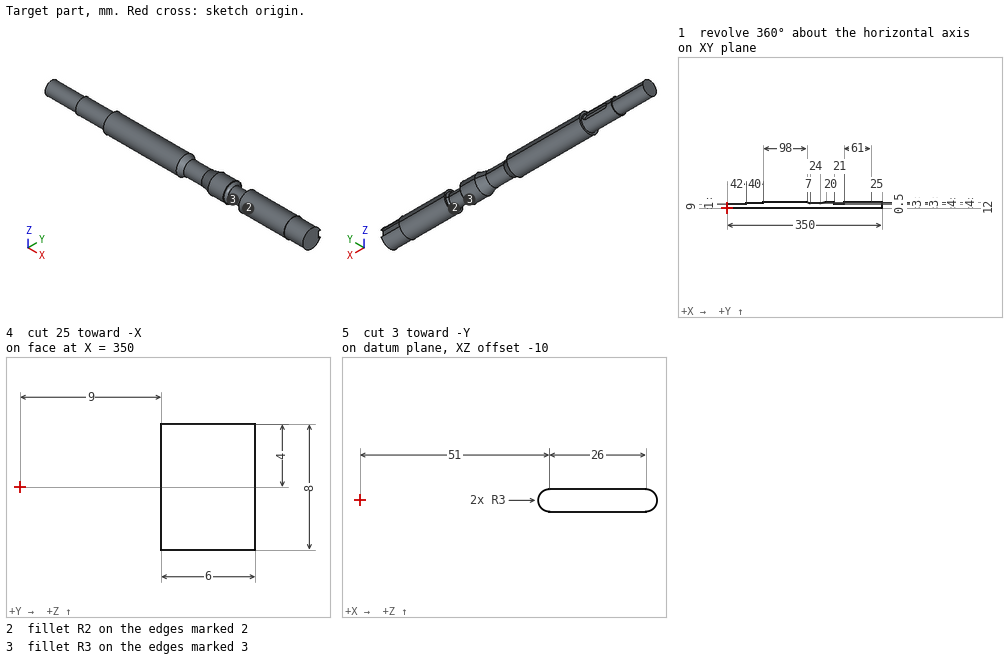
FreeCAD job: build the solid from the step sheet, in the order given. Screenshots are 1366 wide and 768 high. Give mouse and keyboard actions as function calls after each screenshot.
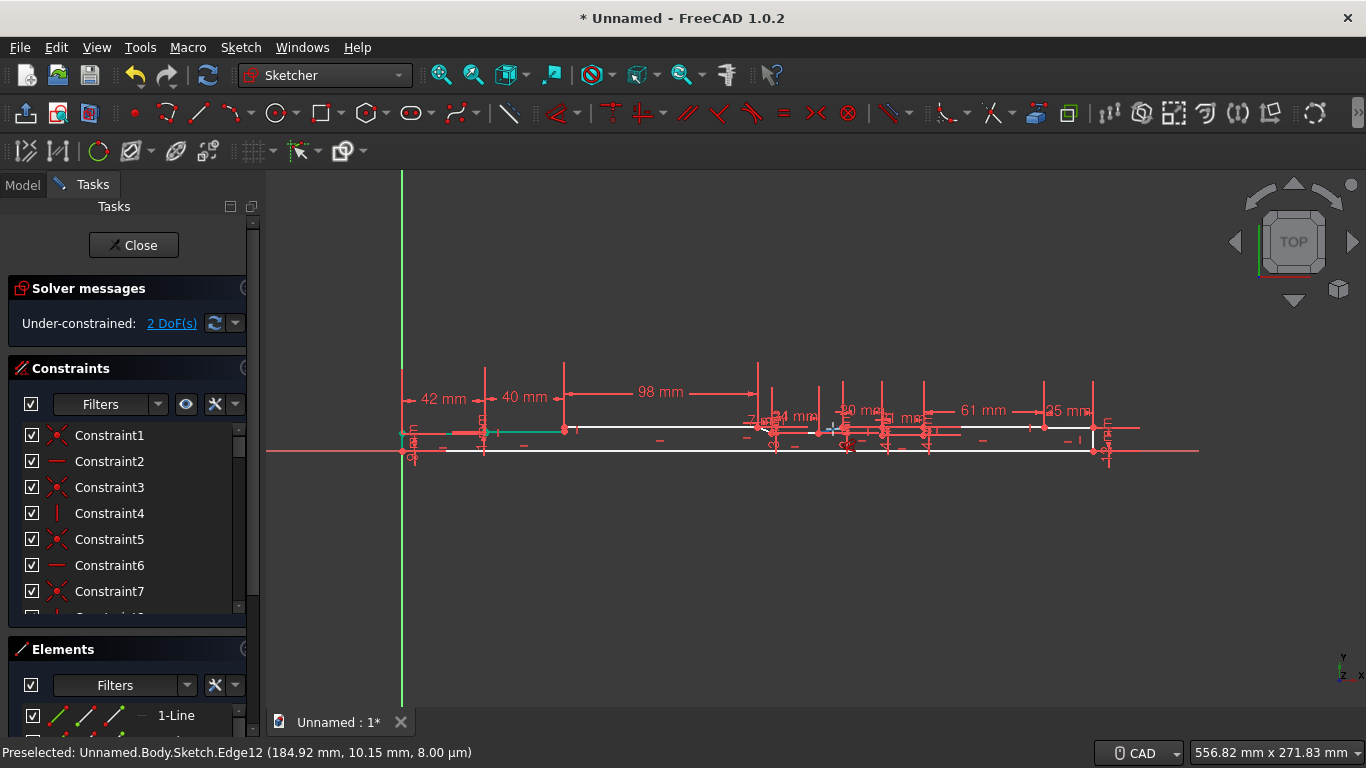
click(817, 451)
click(748, 485)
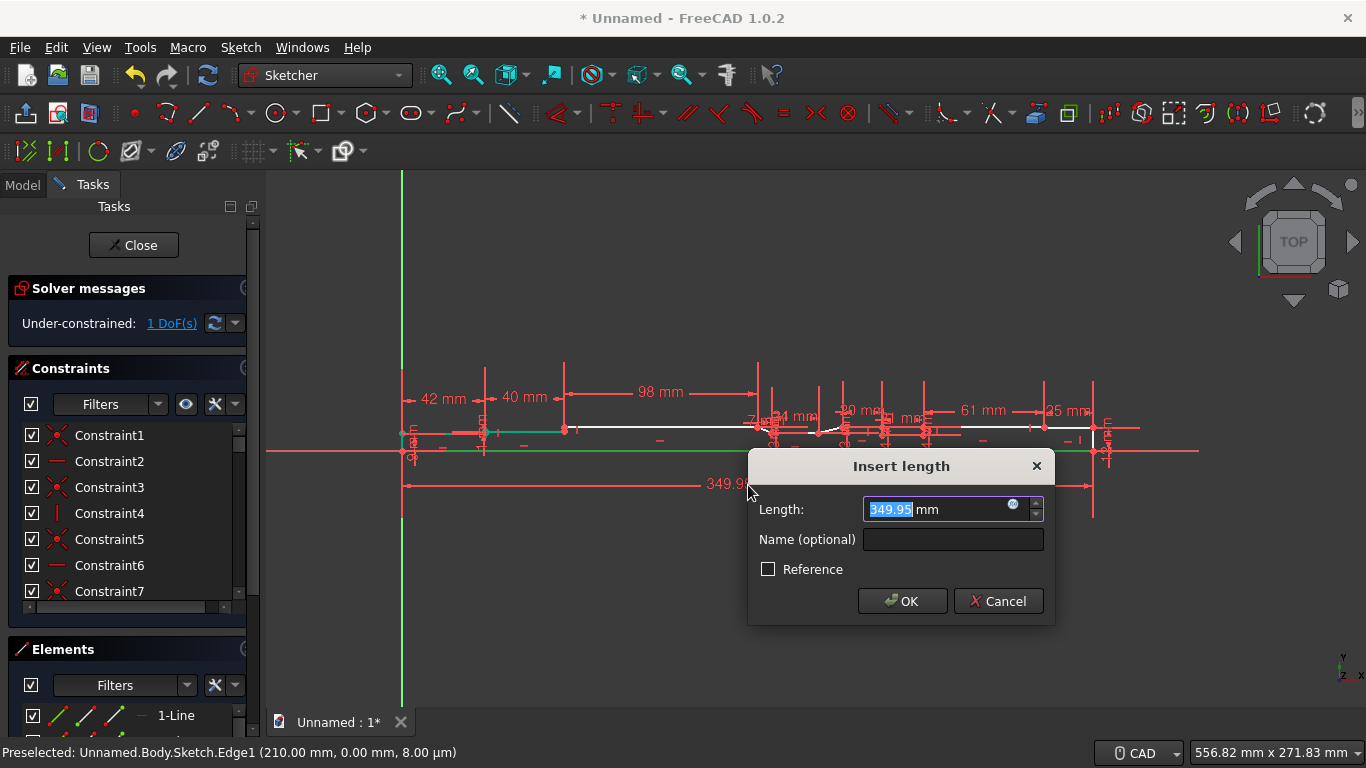
text(350)
key(Return)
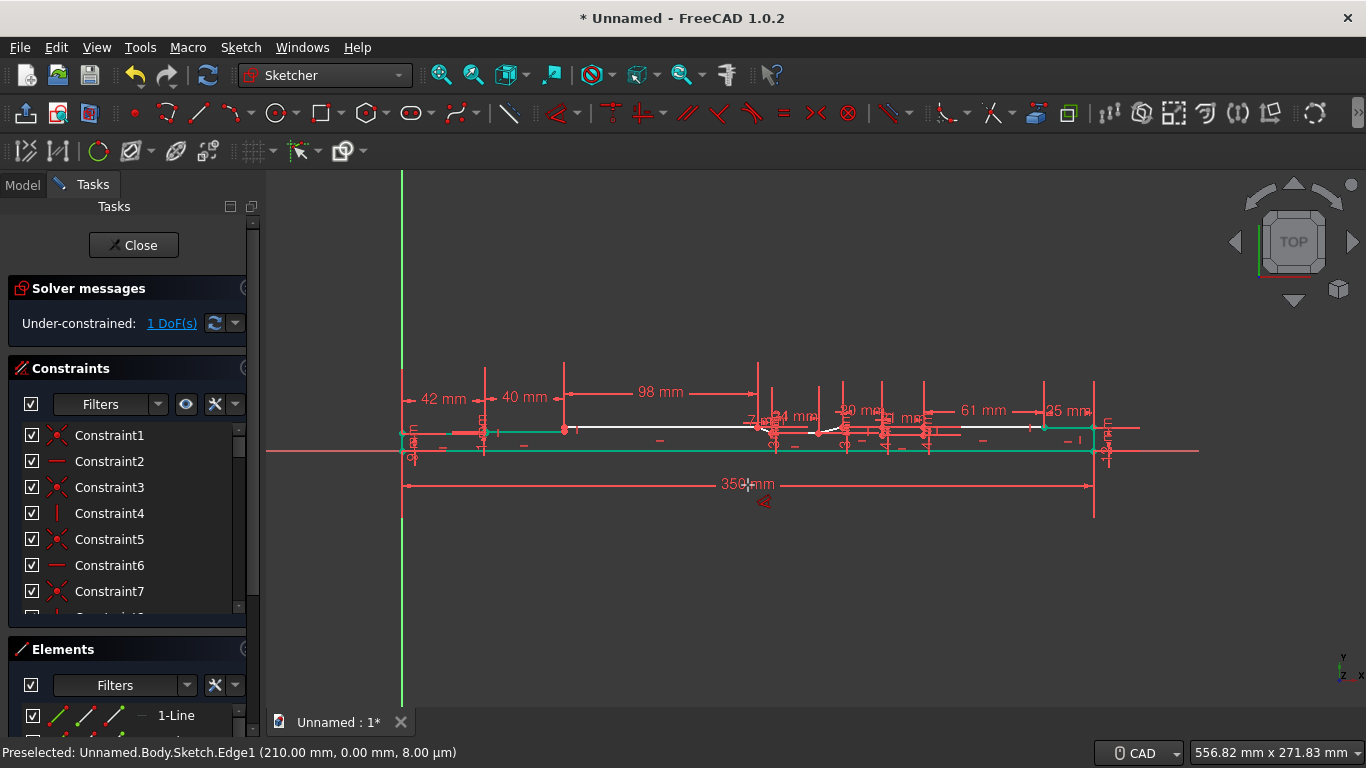
scroll(1044, 427, up, 19)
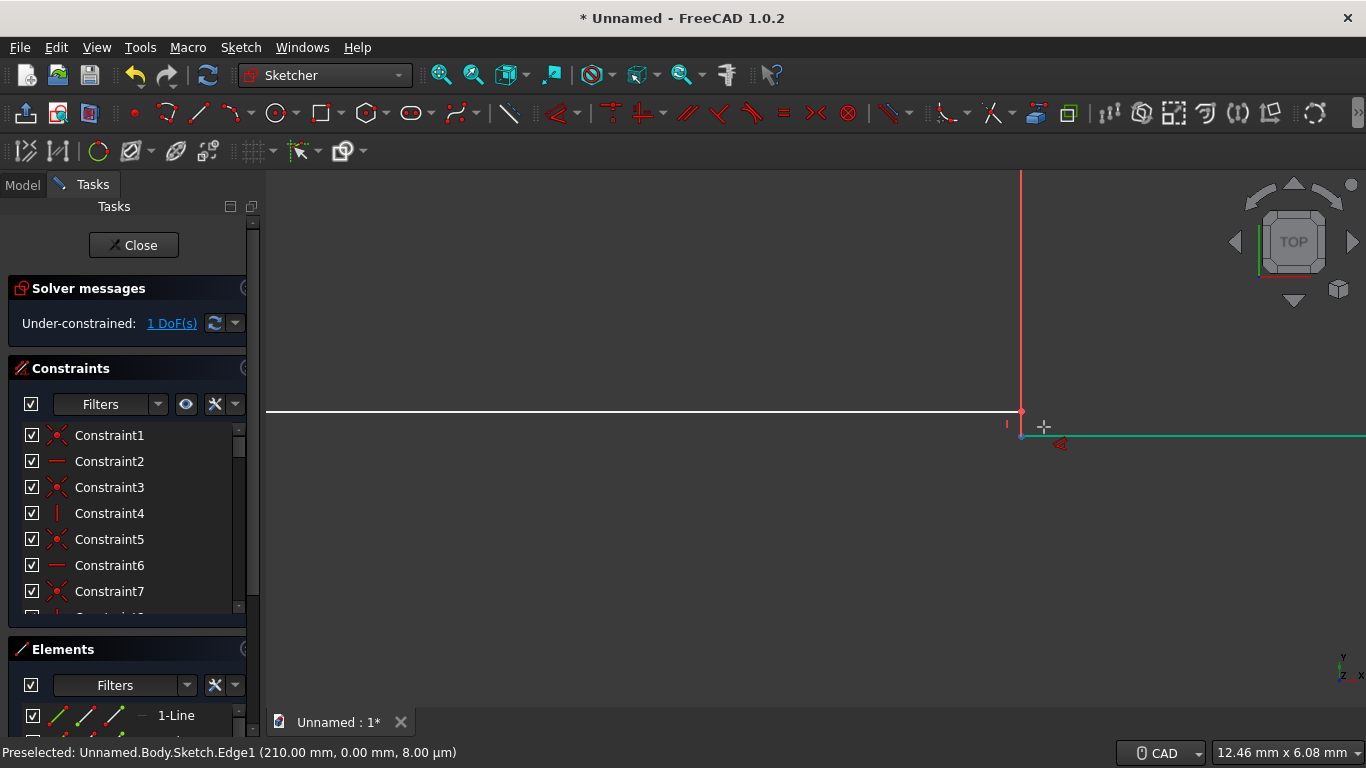
click(1021, 424)
click(1055, 418)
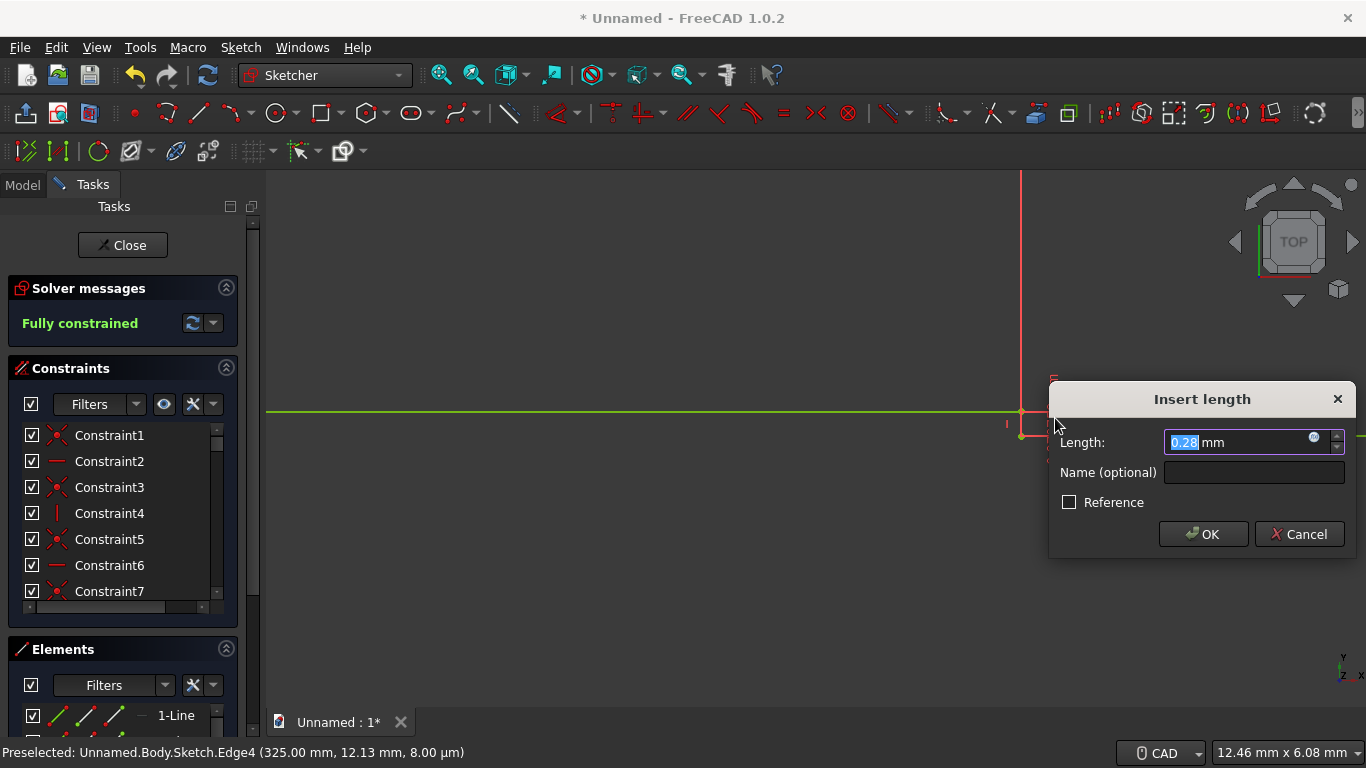
text(0.5)
key(Return)
key(Escape)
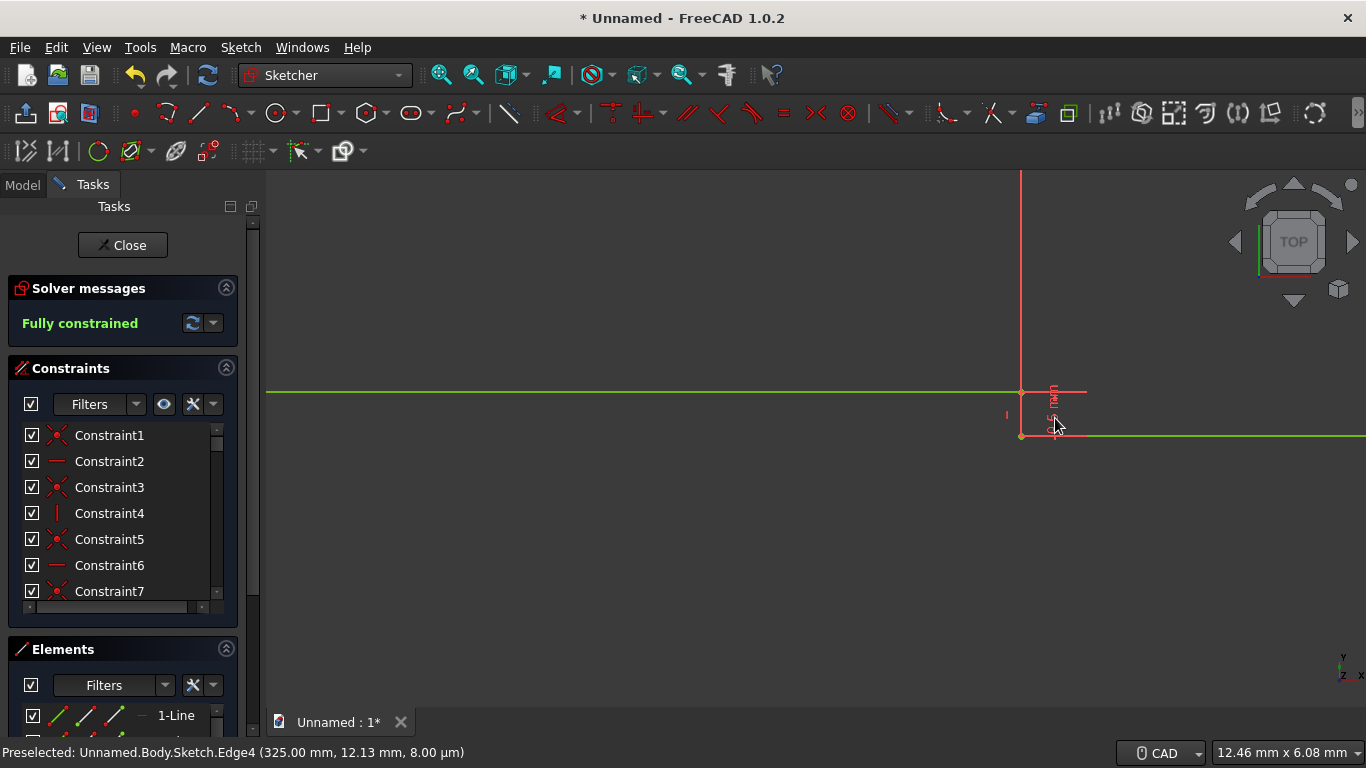
click(123, 245)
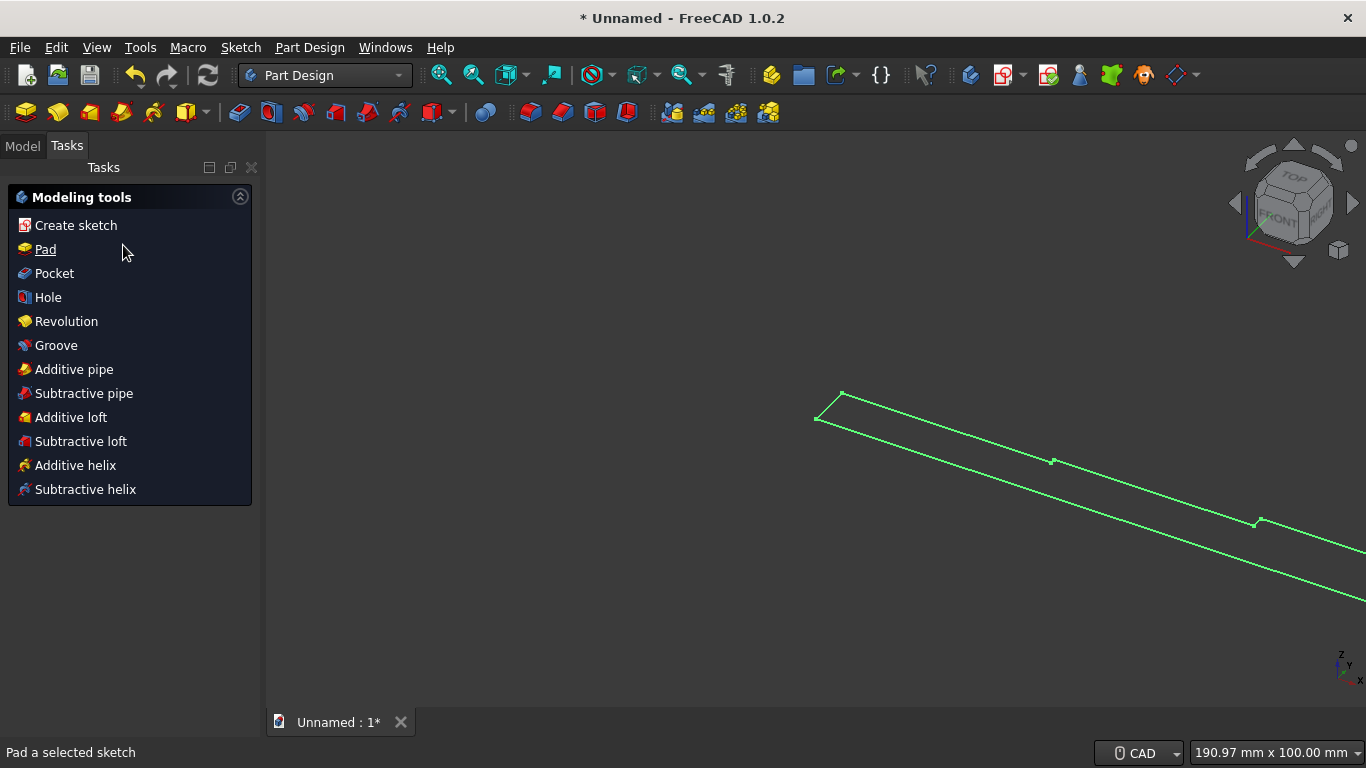
click(58, 112)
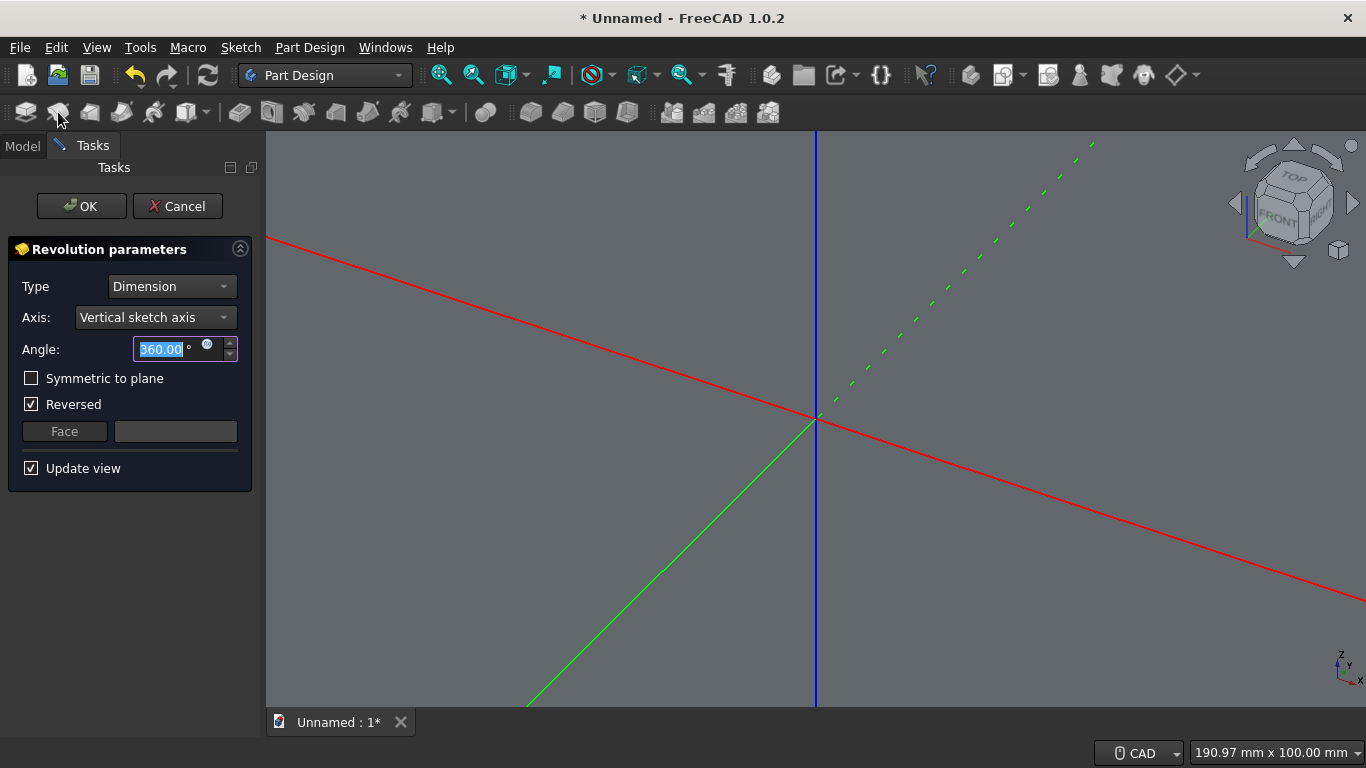
click(156, 318)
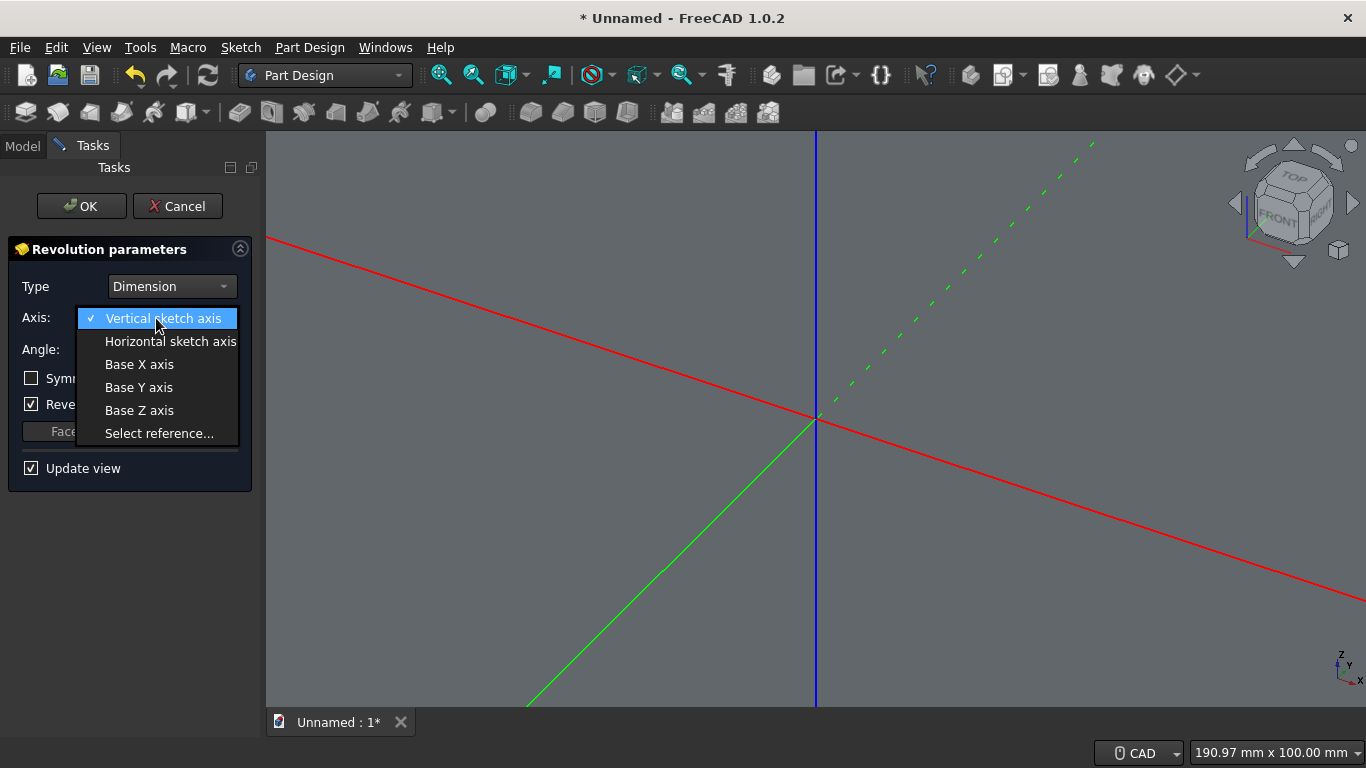
click(156, 342)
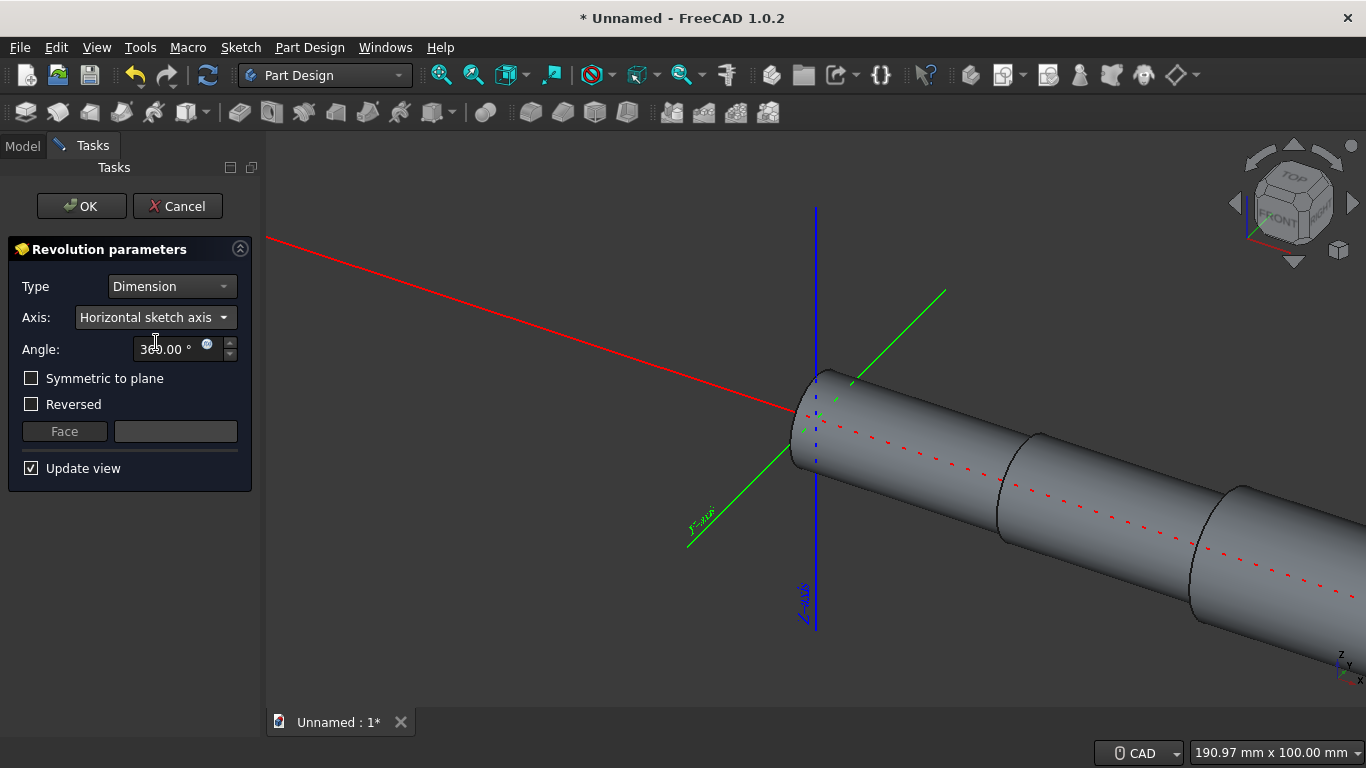
click(82, 206)